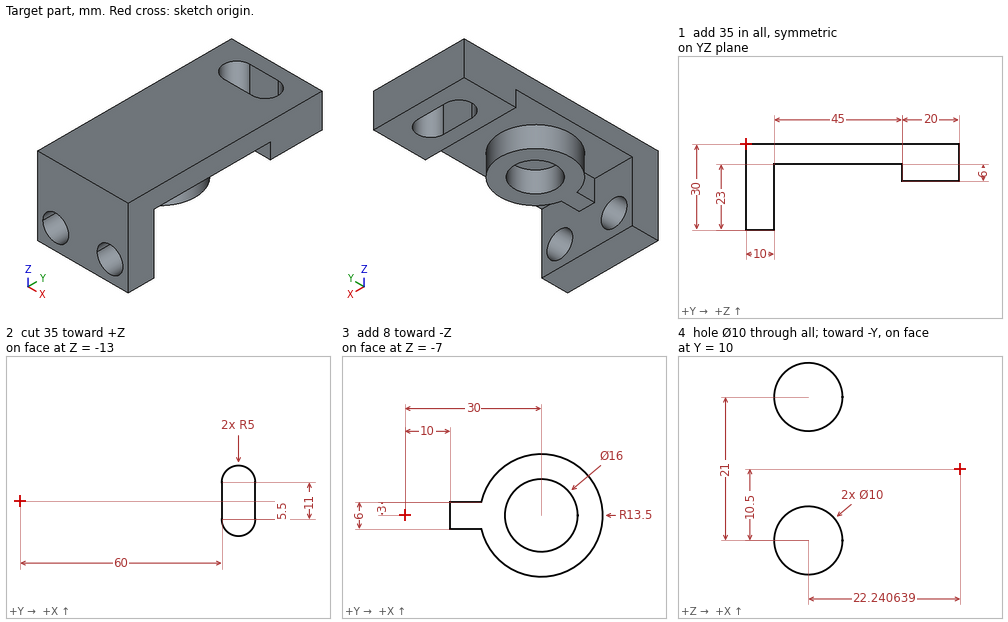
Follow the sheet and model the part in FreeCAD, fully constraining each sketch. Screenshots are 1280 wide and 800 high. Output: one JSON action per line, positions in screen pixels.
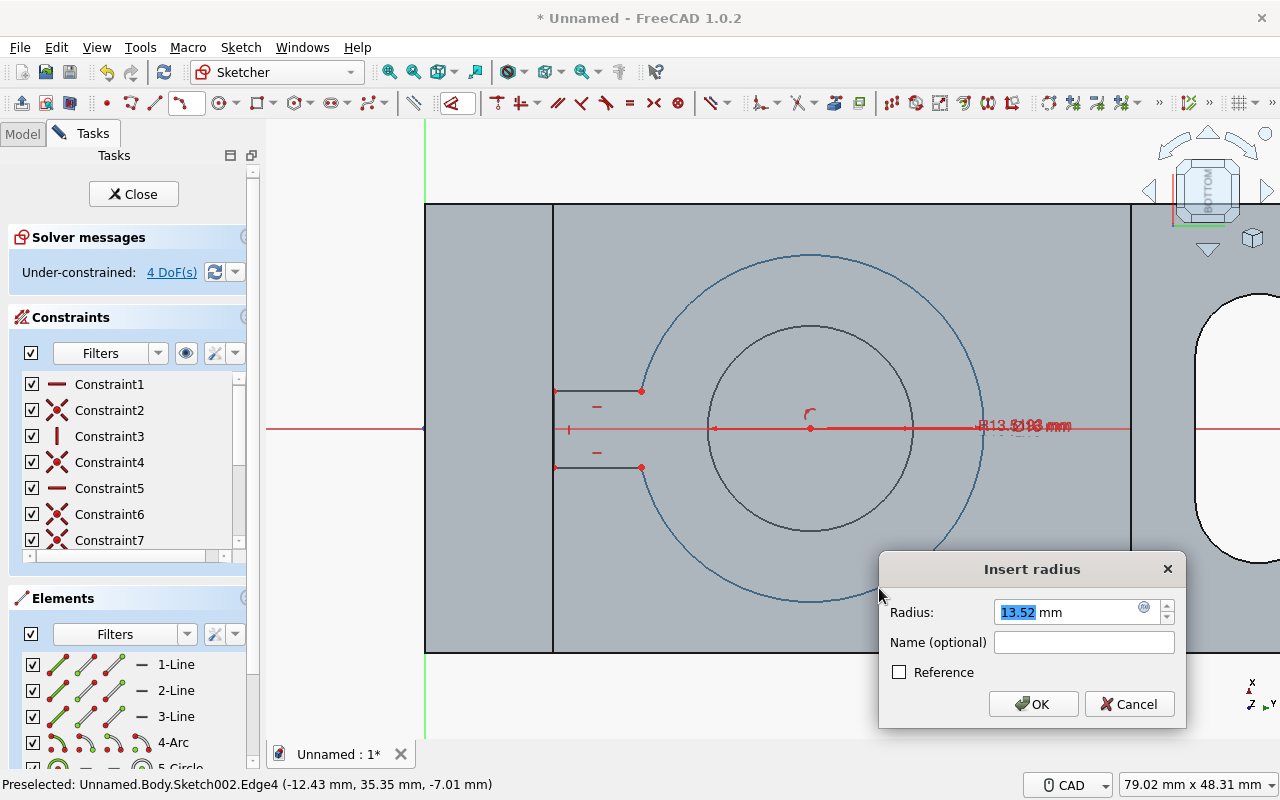
{"action": "type", "text": "13.5"}
{"action": "key", "text": "Return"}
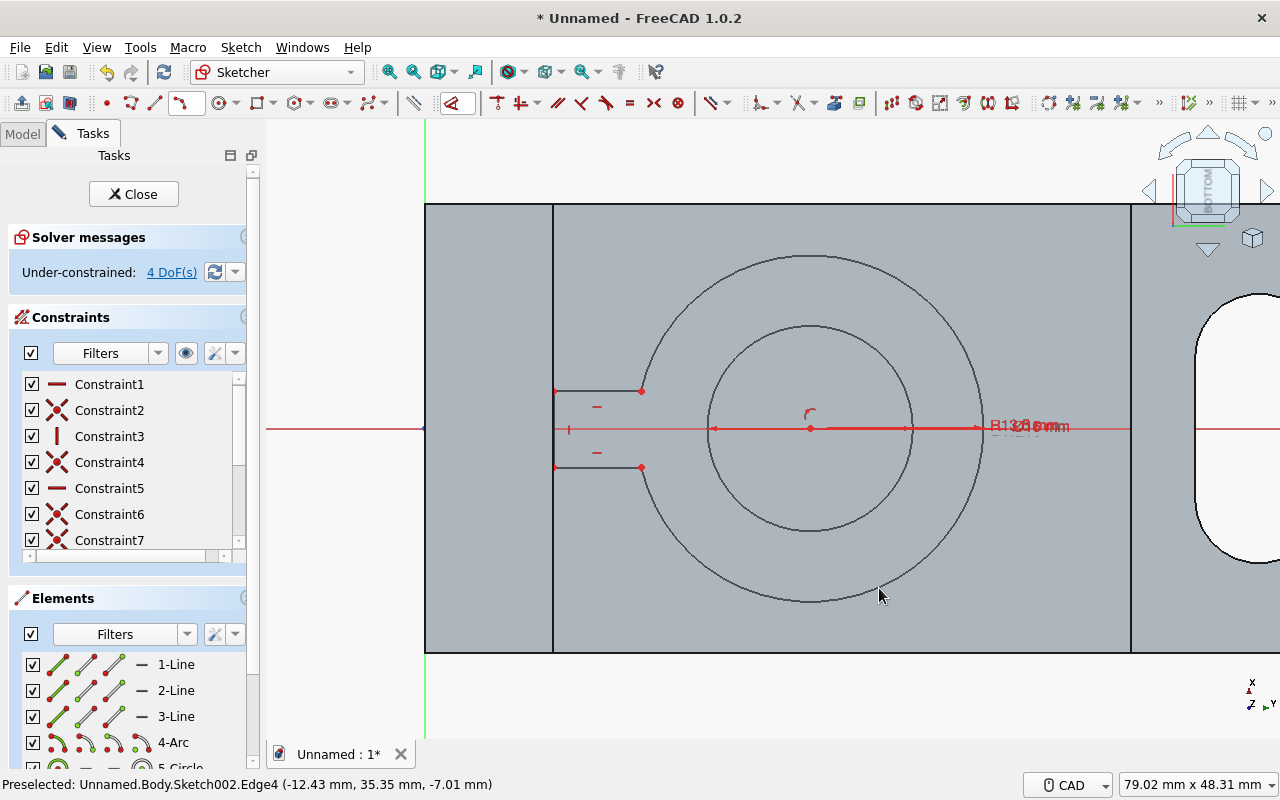
{"action": "left_click", "coordinate": [554, 414]}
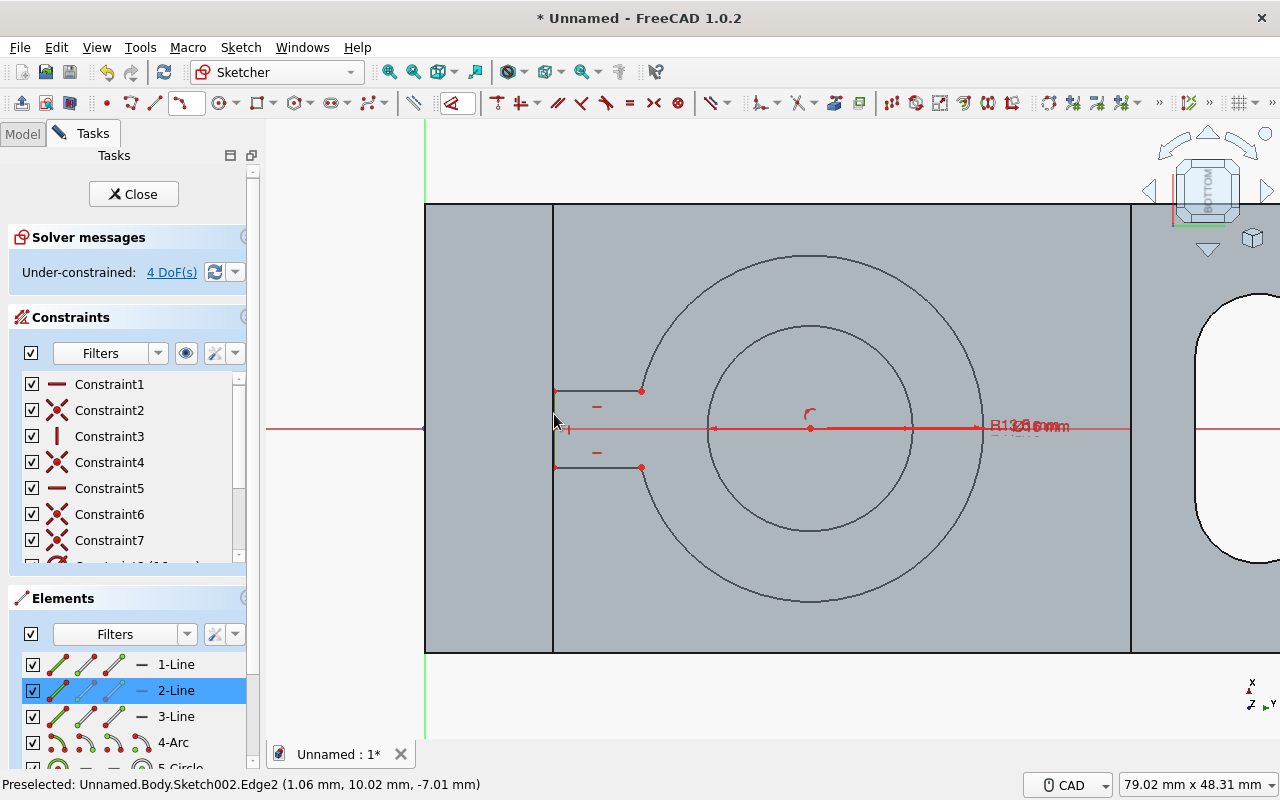
{"action": "left_click", "coordinate": [470, 104]}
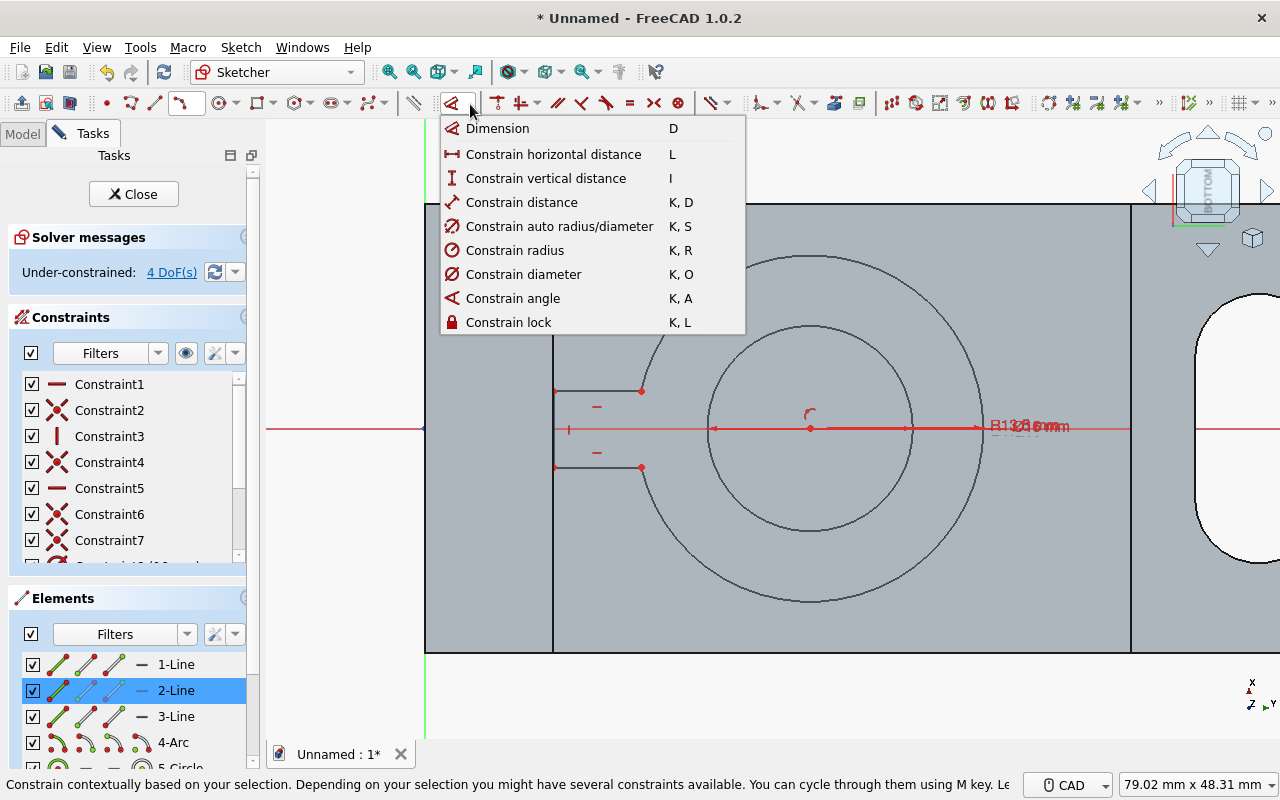
{"action": "left_click", "coordinate": [593, 178]}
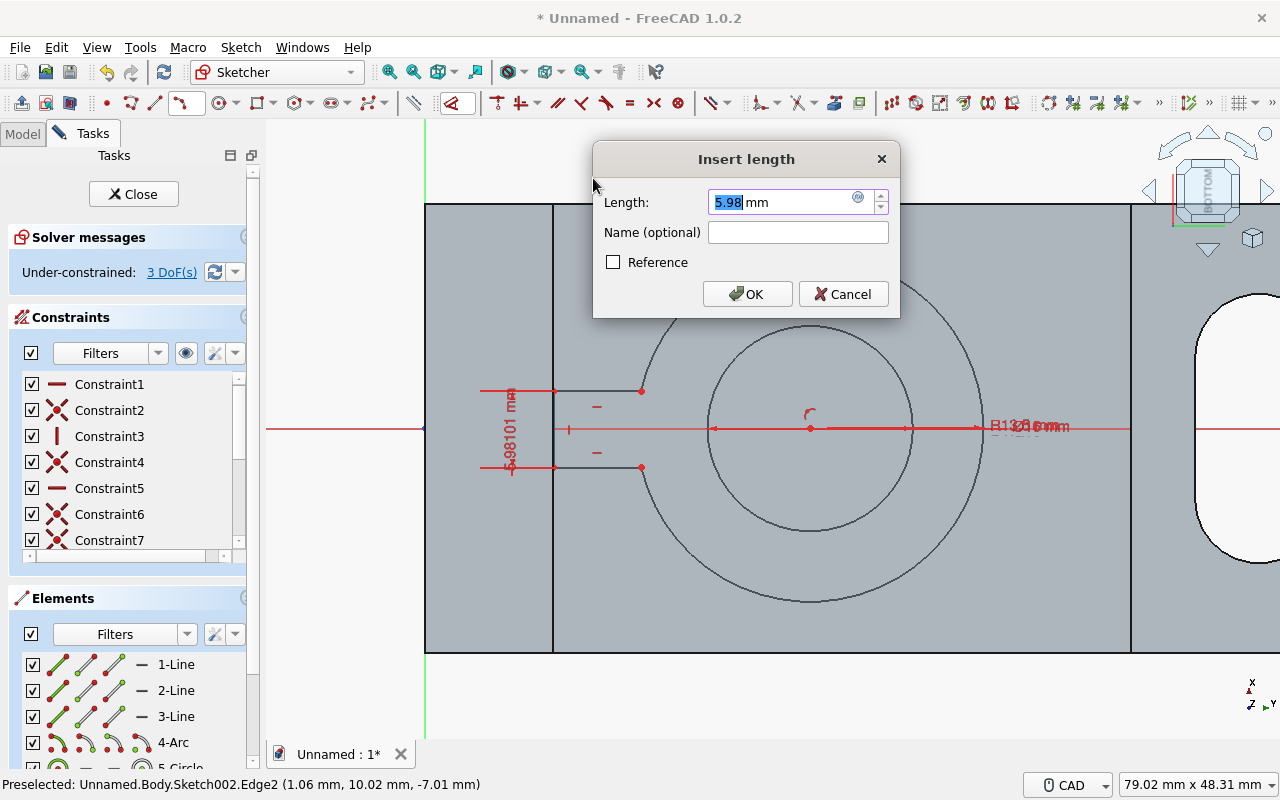
{"action": "type", "text": "6"}
{"action": "key", "text": "Return"}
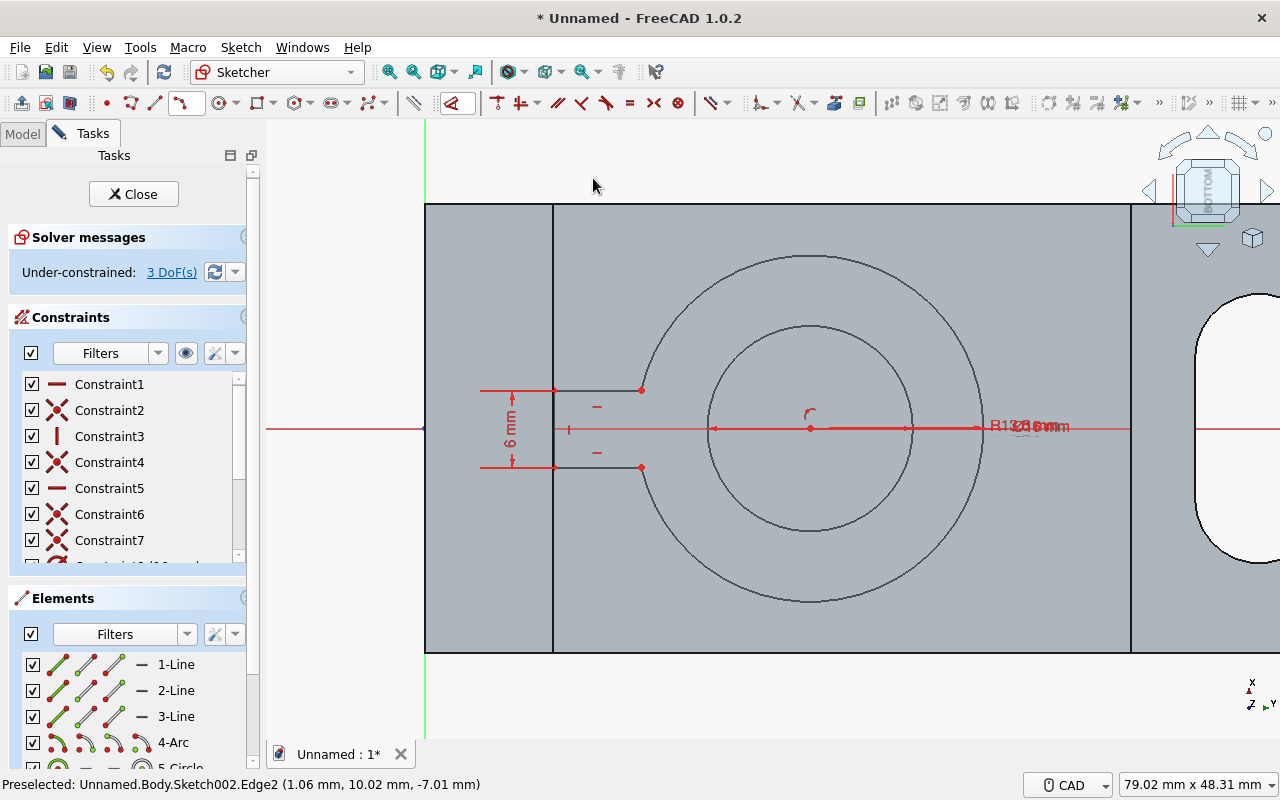
{"action": "left_click", "coordinate": [641, 391]}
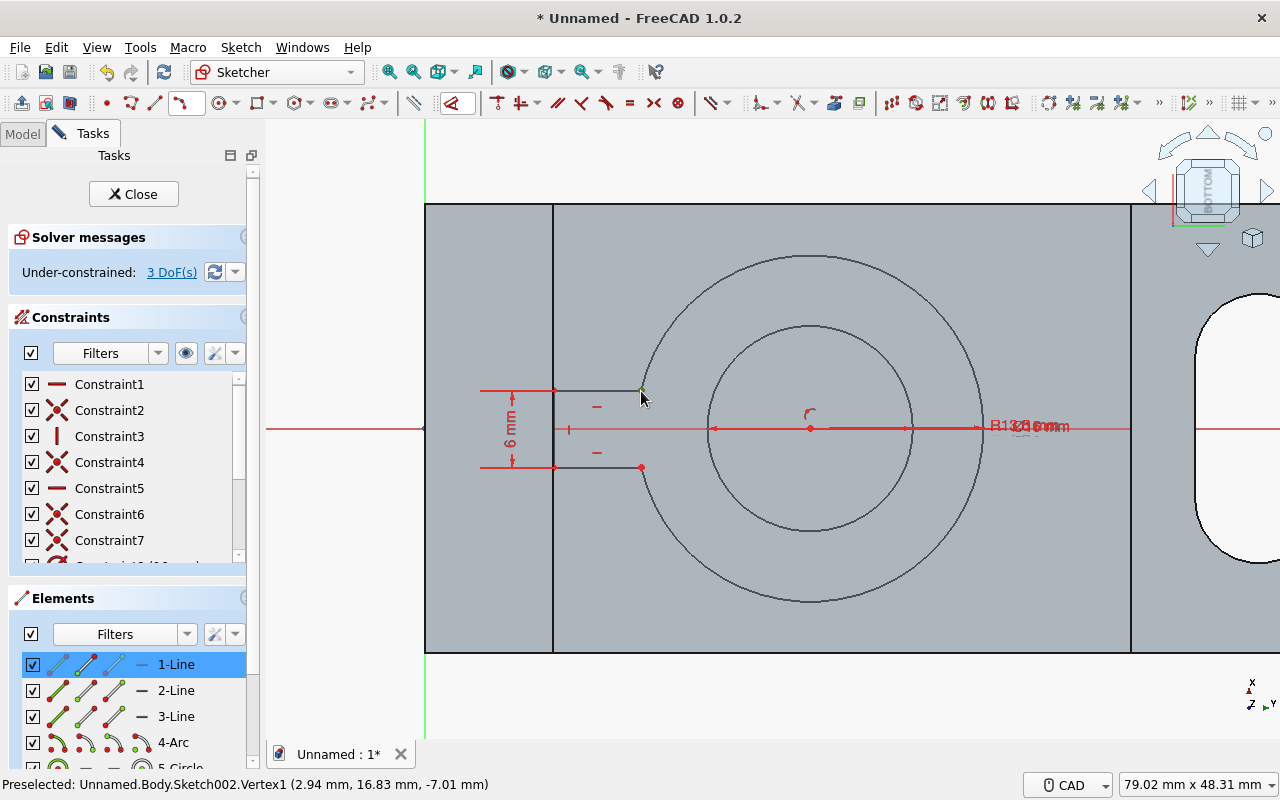
{"action": "left_click", "coordinate": [470, 104]}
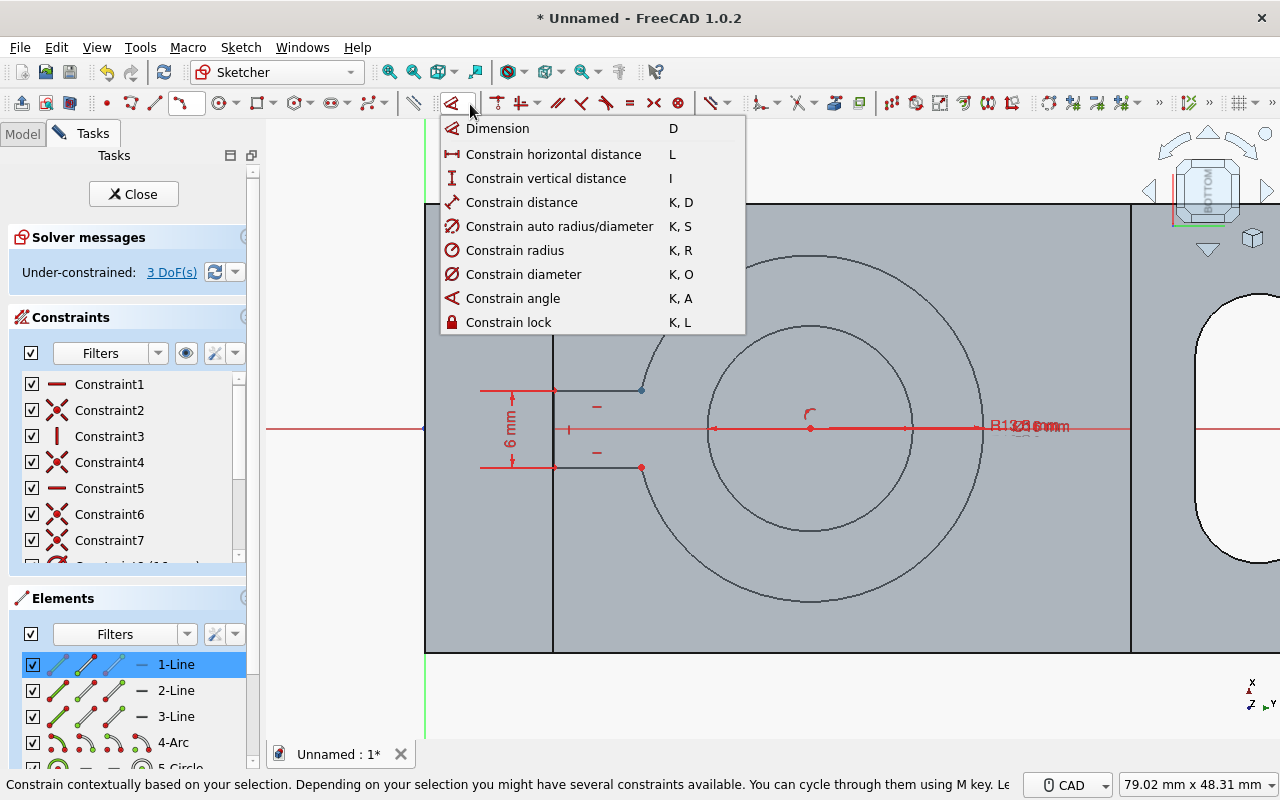
{"action": "left_click", "coordinate": [593, 178]}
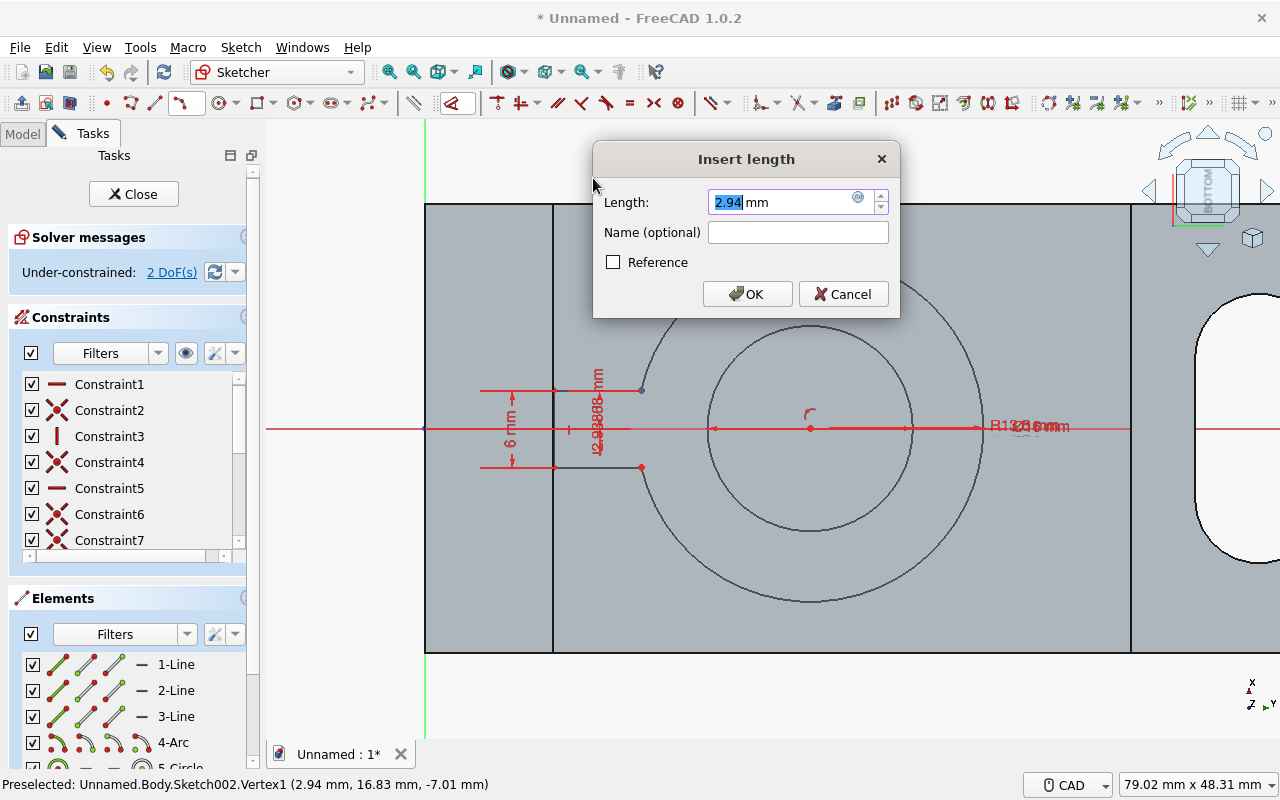
{"action": "type", "text": "3"}
{"action": "key", "text": "Return"}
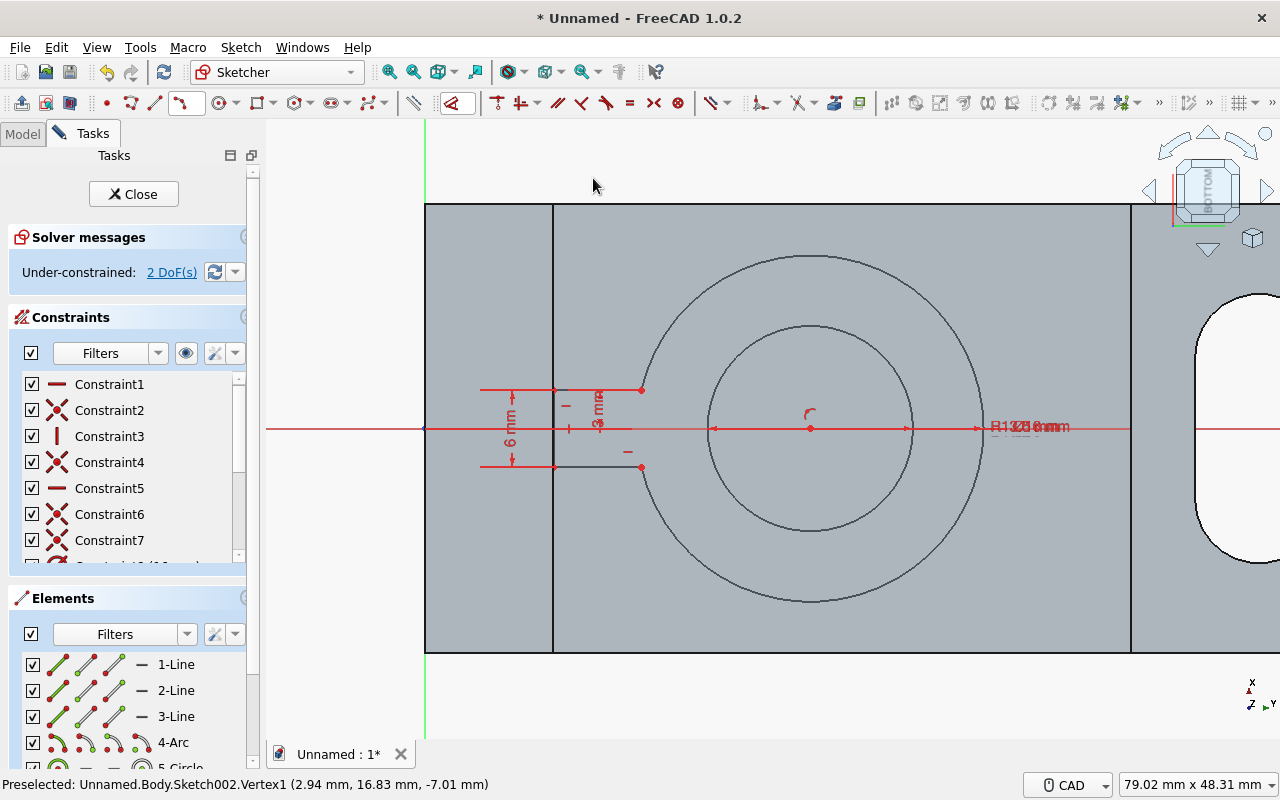
{"action": "left_click", "coordinate": [810, 429]}